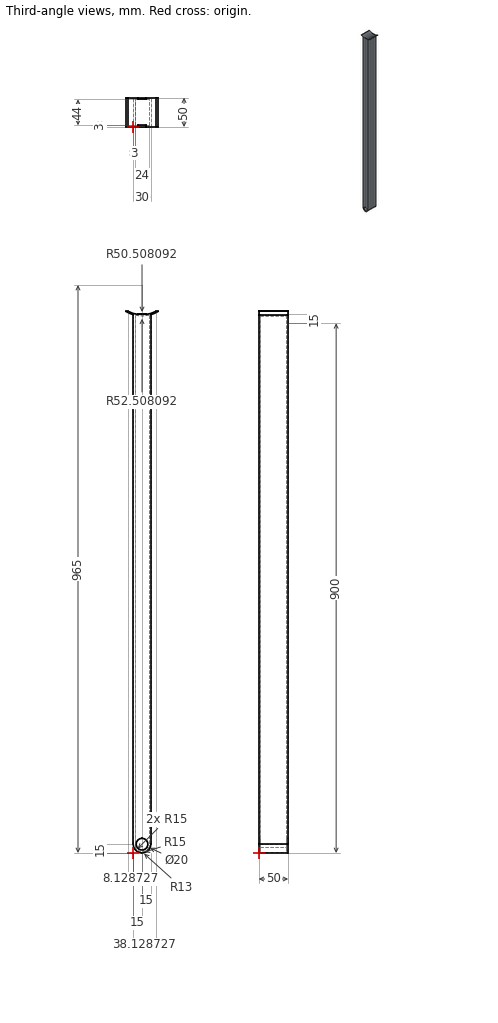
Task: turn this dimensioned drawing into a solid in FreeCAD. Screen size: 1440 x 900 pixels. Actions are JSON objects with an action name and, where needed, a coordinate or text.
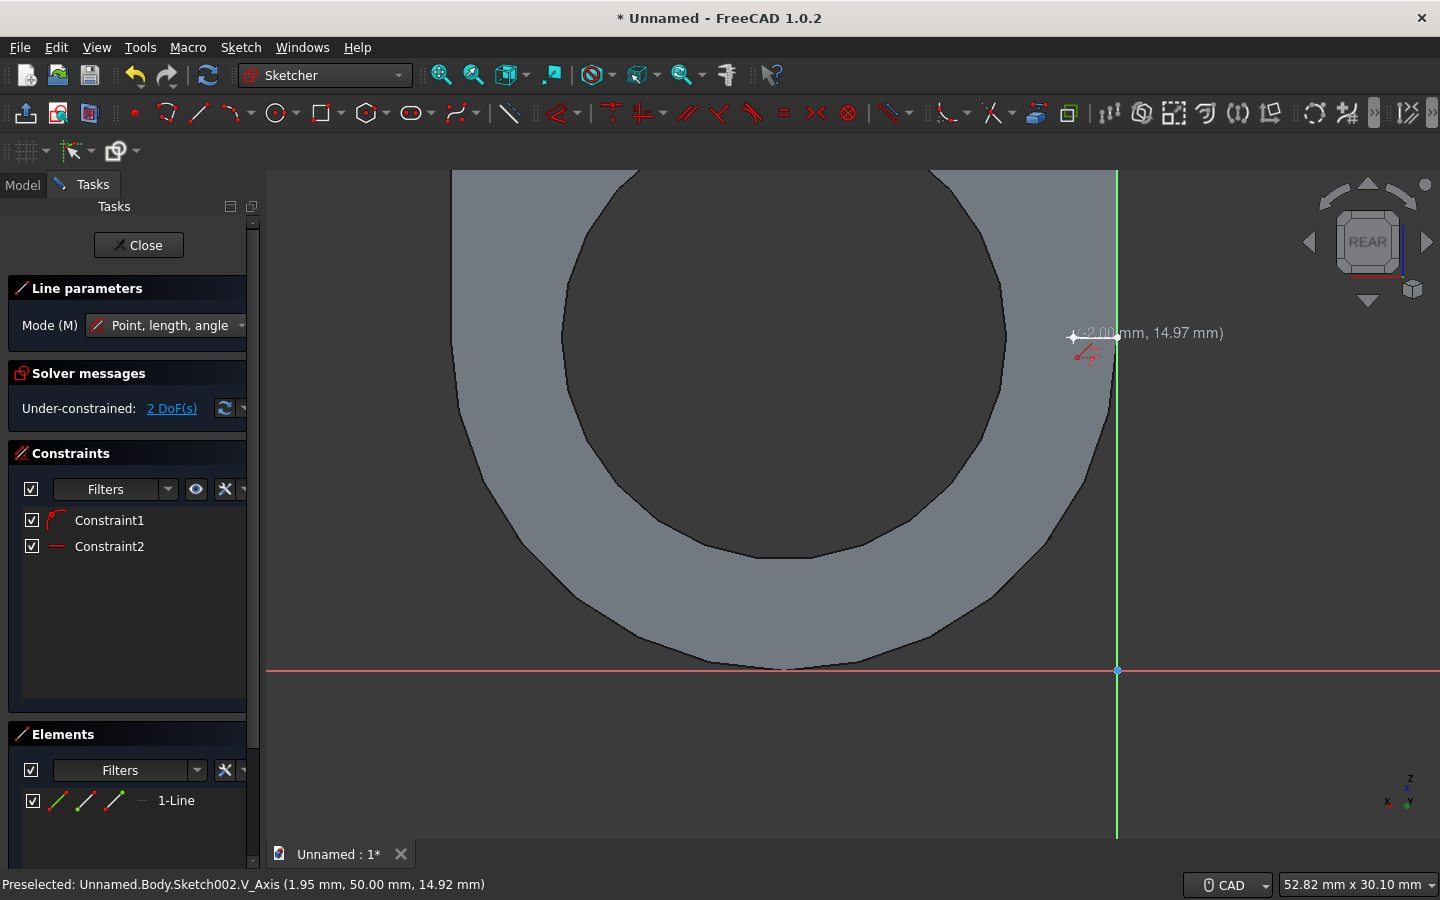
{"action": "left_click", "coordinate": [495, 337]}
{"action": "left_click", "coordinate": [451, 337]}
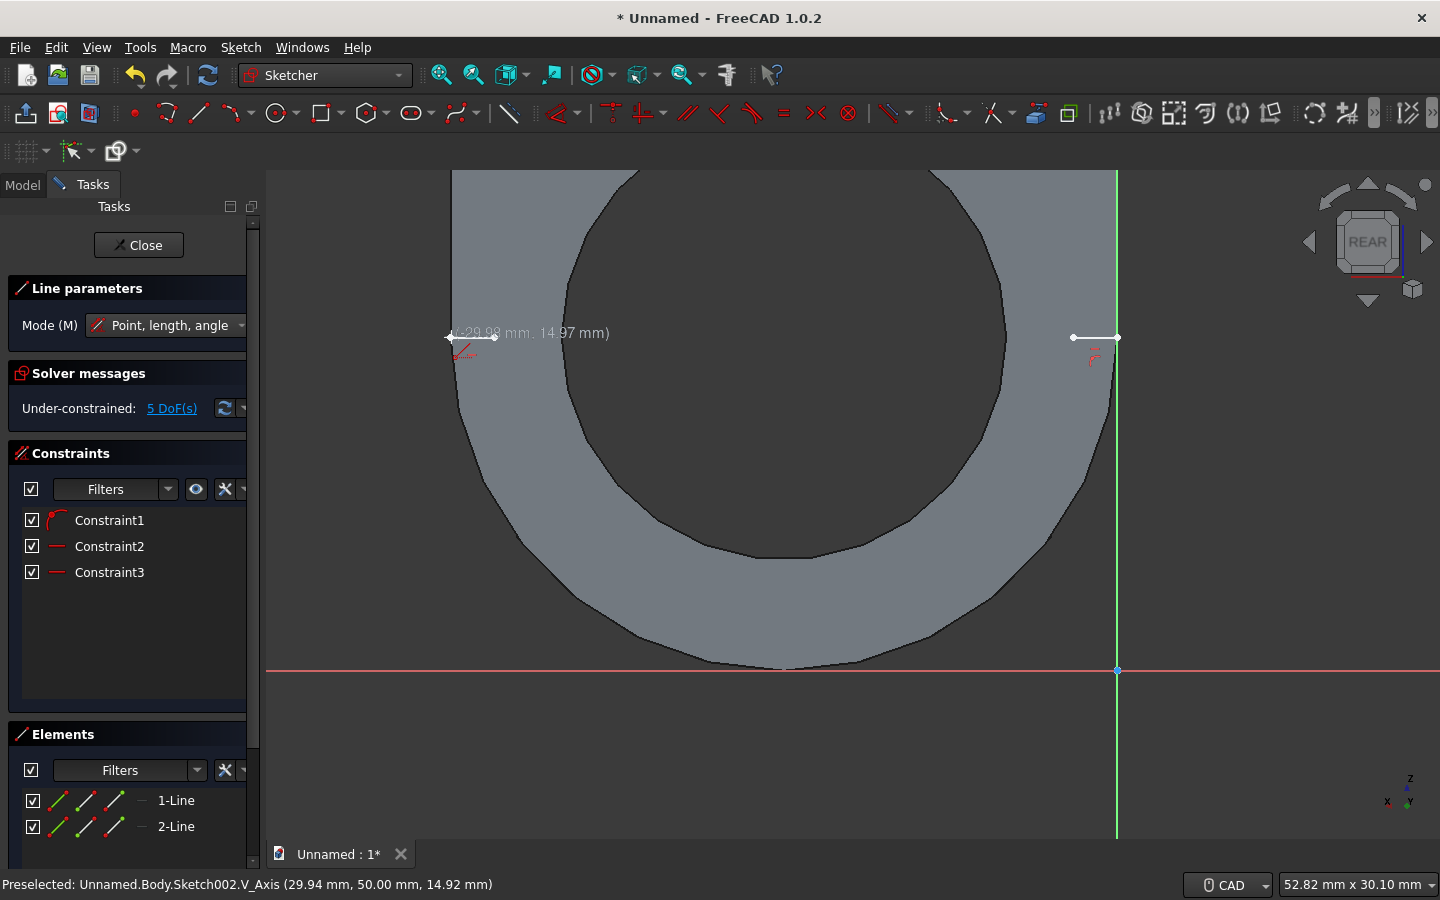
{"action": "left_click", "coordinate": [232, 114]}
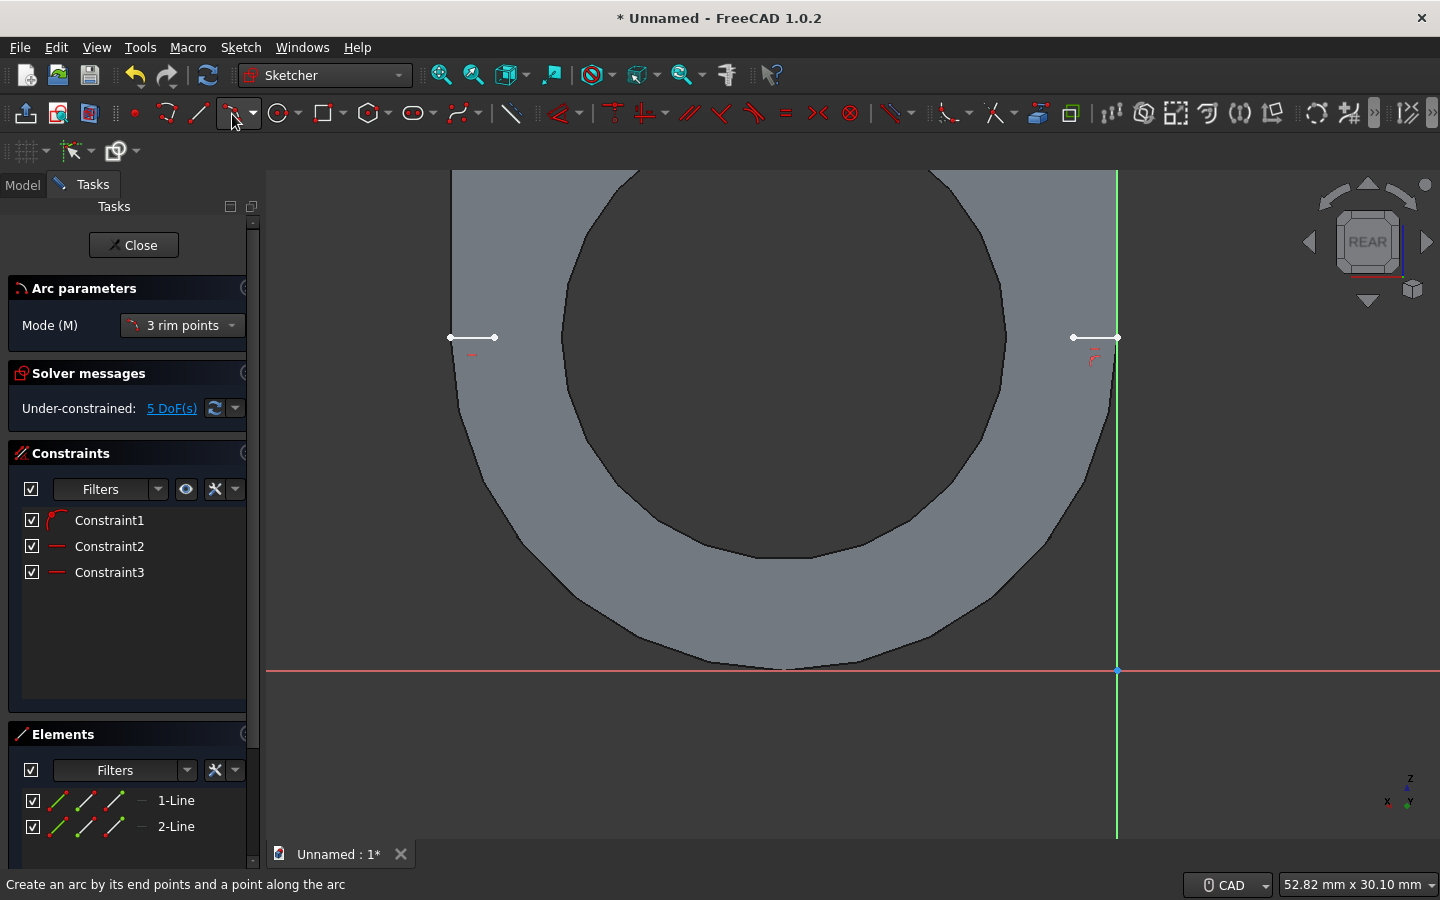
{"action": "left_click", "coordinate": [1073, 338]}
{"action": "left_click", "coordinate": [495, 338]}
{"action": "left_click", "coordinate": [784, 626]}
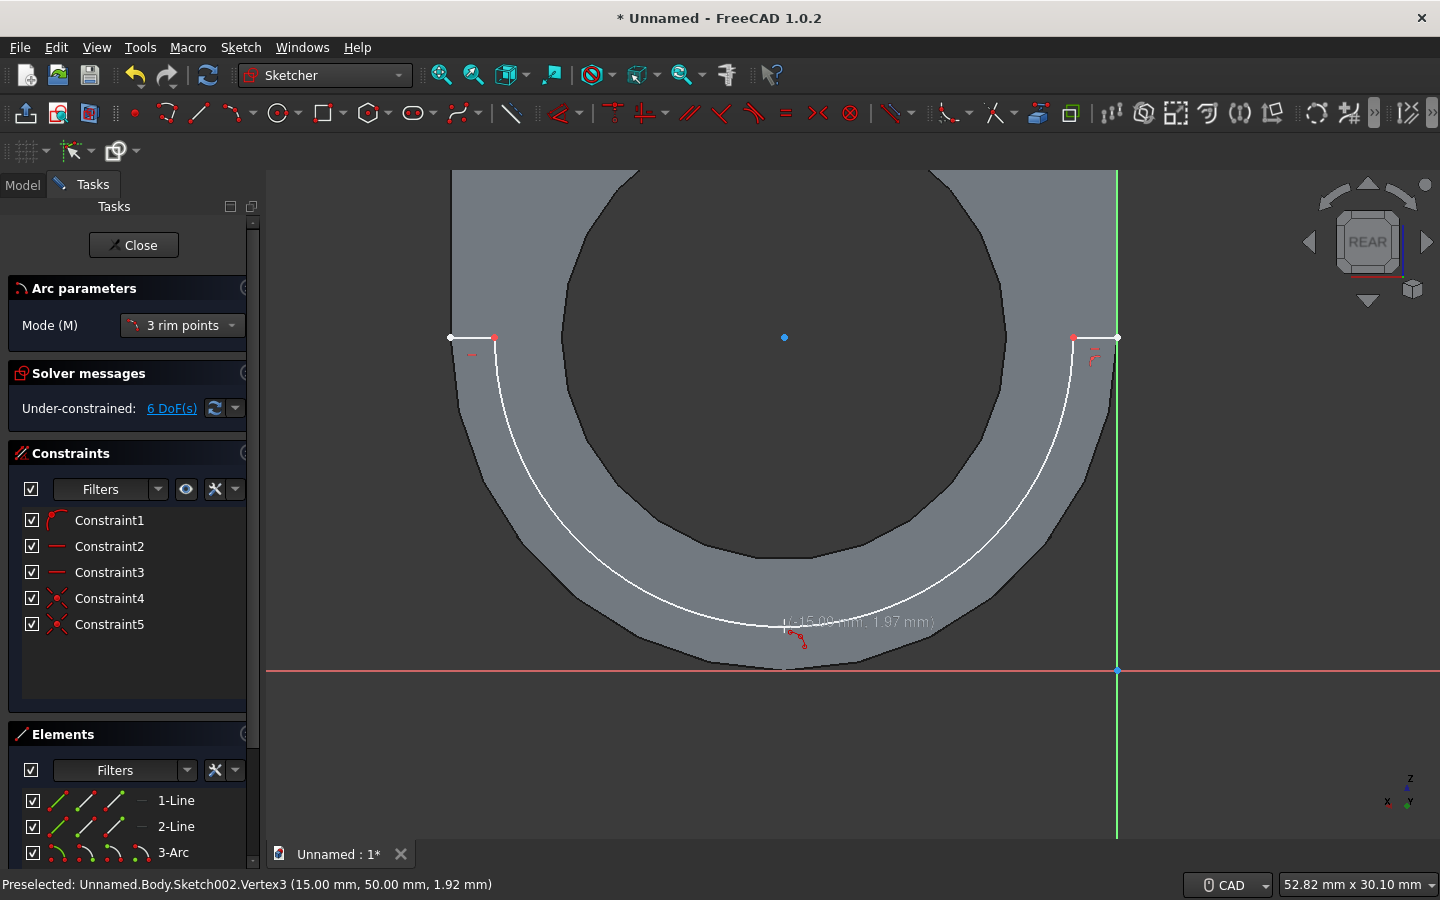
{"action": "left_click", "coordinate": [451, 338]}
{"action": "left_click", "coordinate": [1117, 338]}
{"action": "left_click", "coordinate": [681, 654]}
{"action": "key", "text": "Escape"}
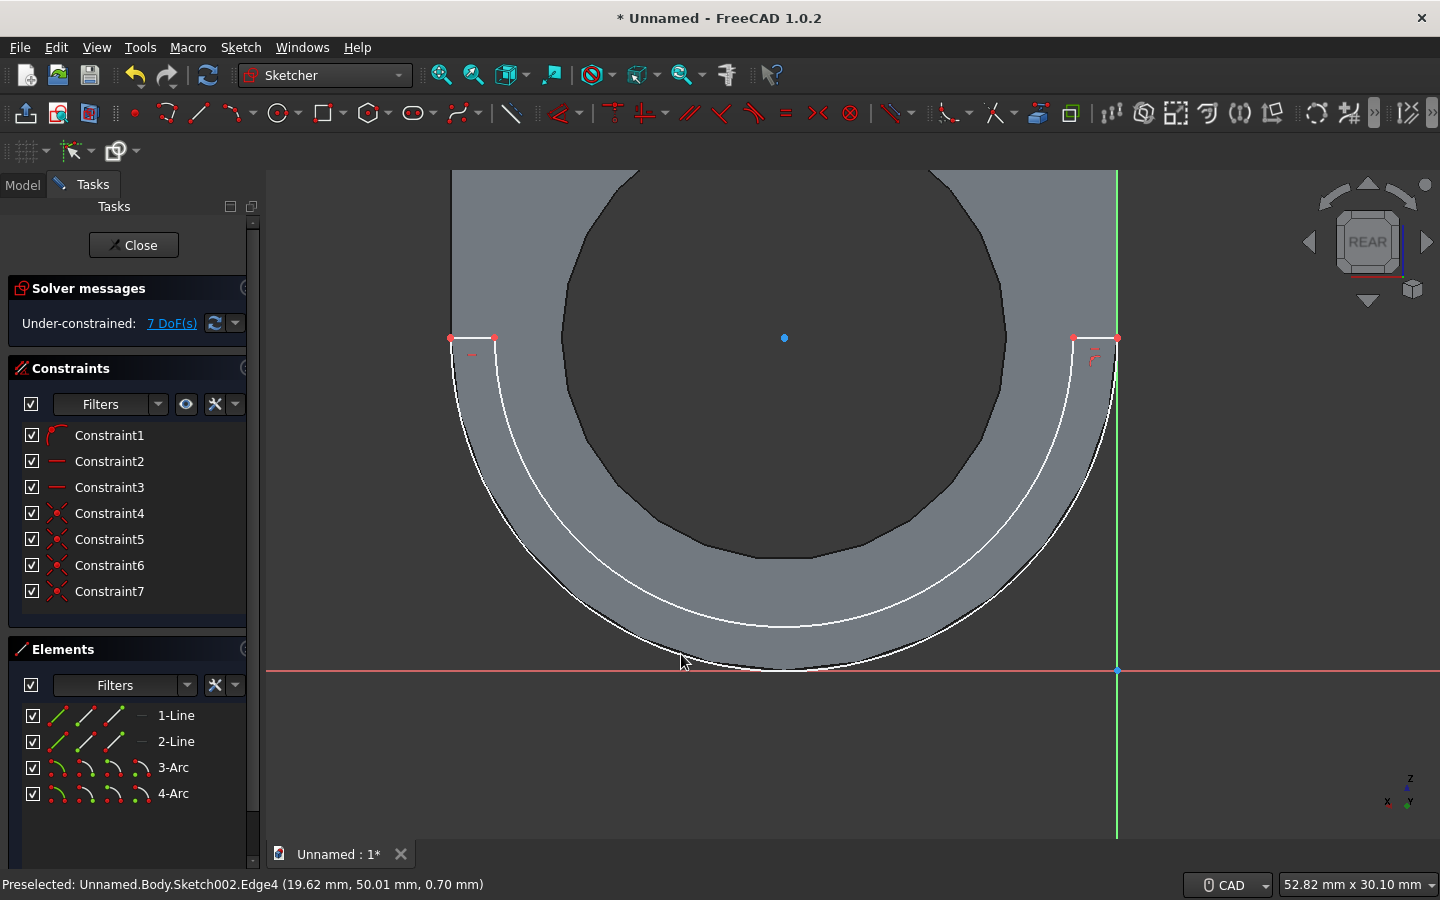
{"action": "left_click", "coordinate": [614, 572]}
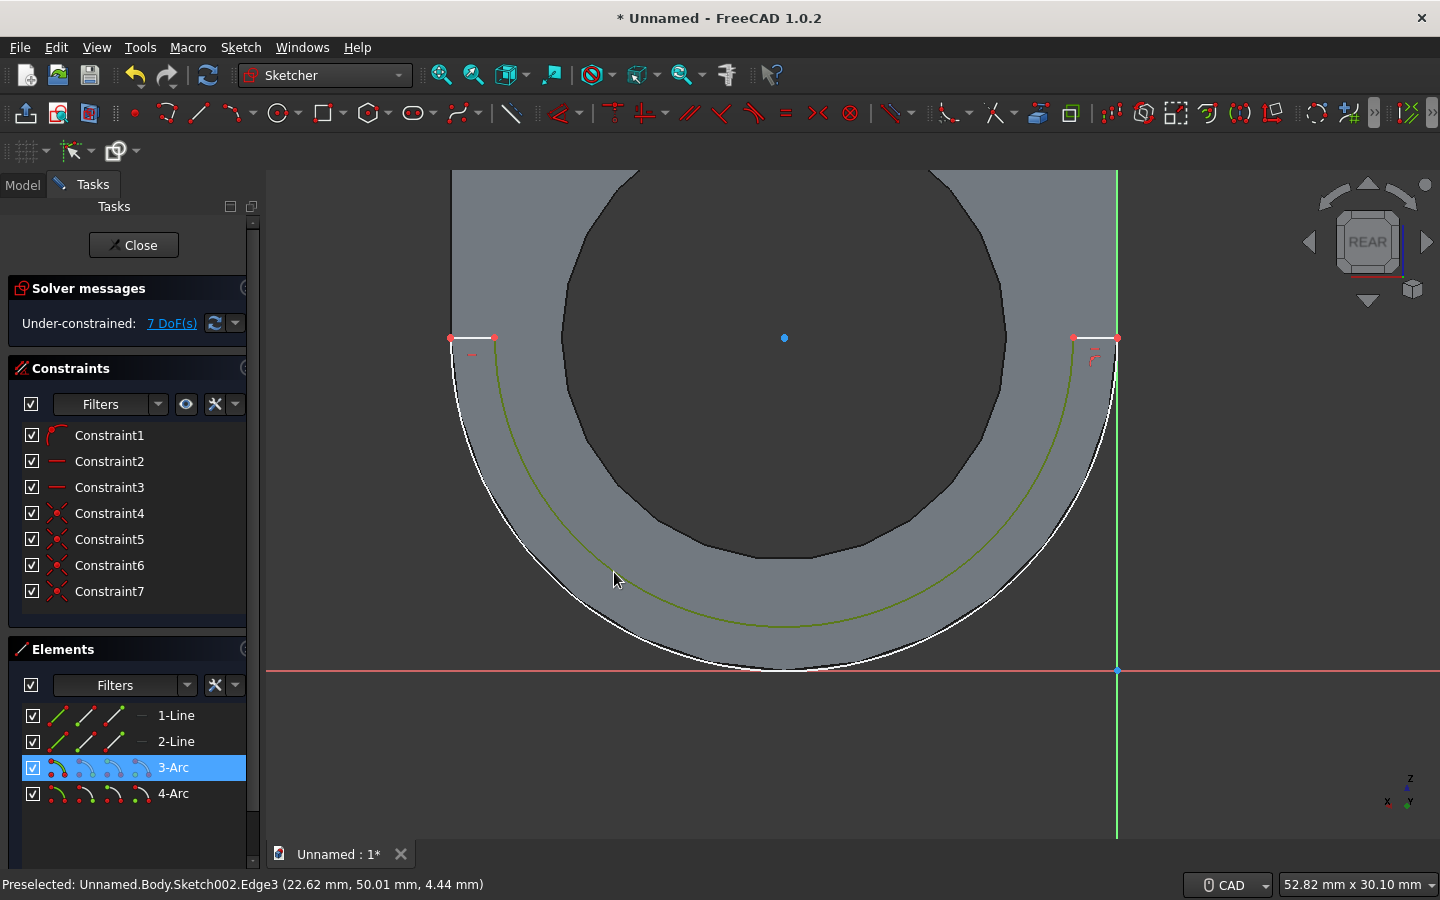
{"action": "left_click", "coordinate": [588, 608]}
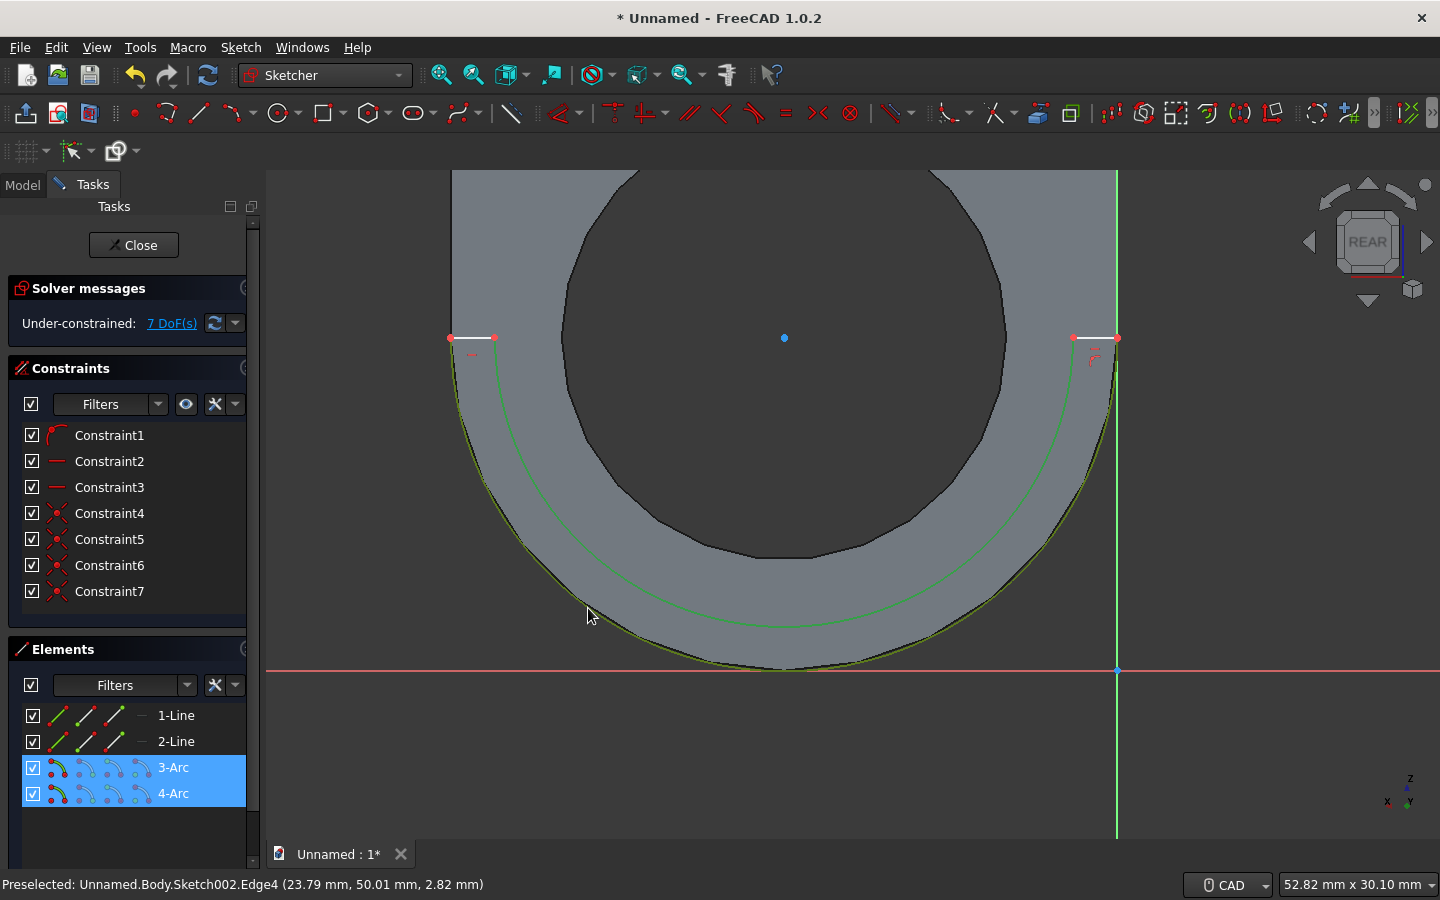
{"action": "left_click", "coordinate": [614, 114]}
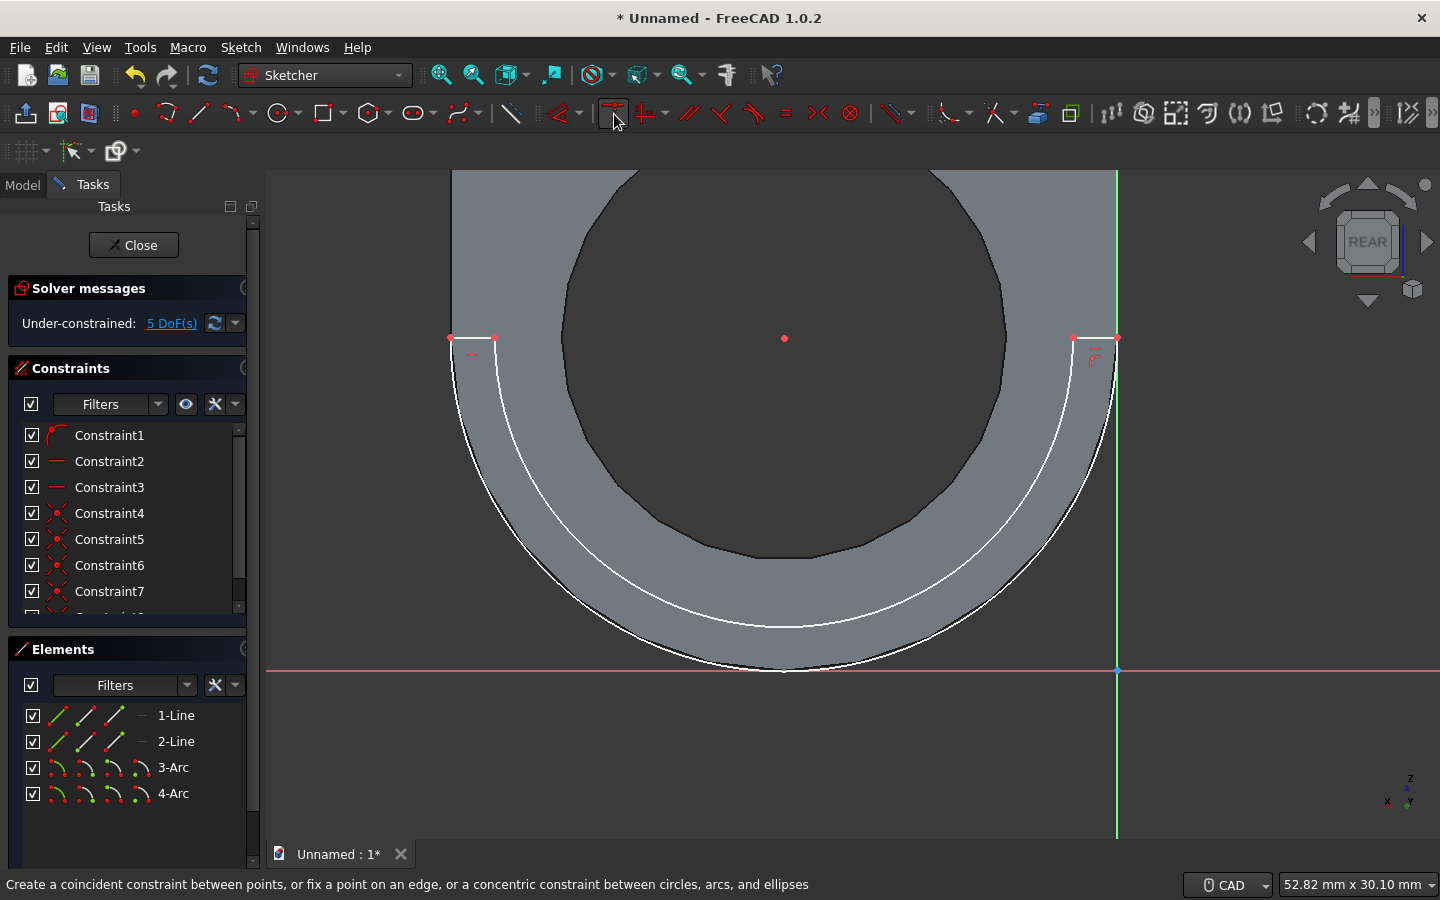
{"action": "left_click", "coordinate": [558, 114]}